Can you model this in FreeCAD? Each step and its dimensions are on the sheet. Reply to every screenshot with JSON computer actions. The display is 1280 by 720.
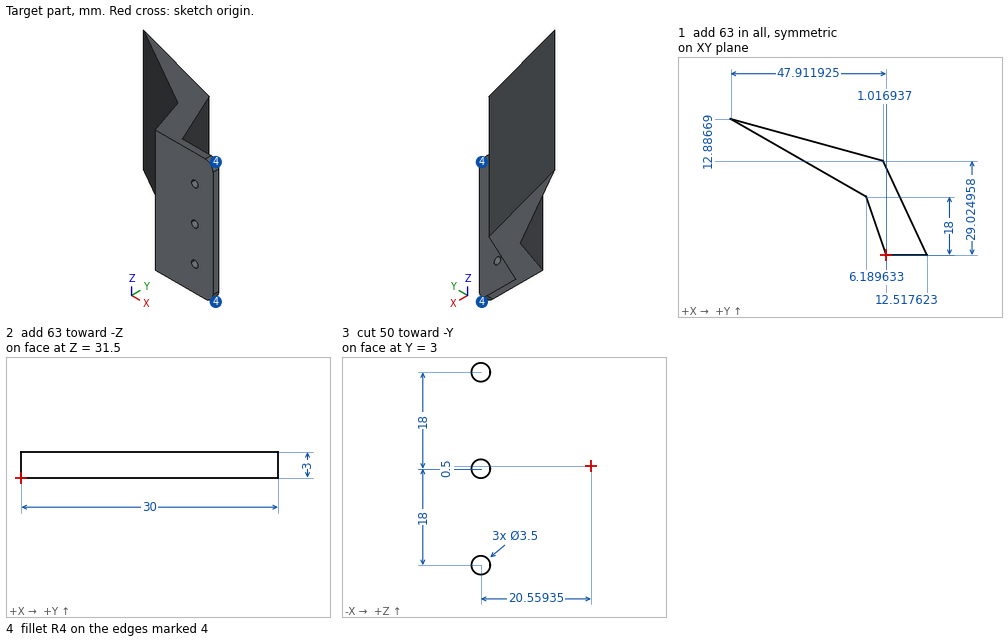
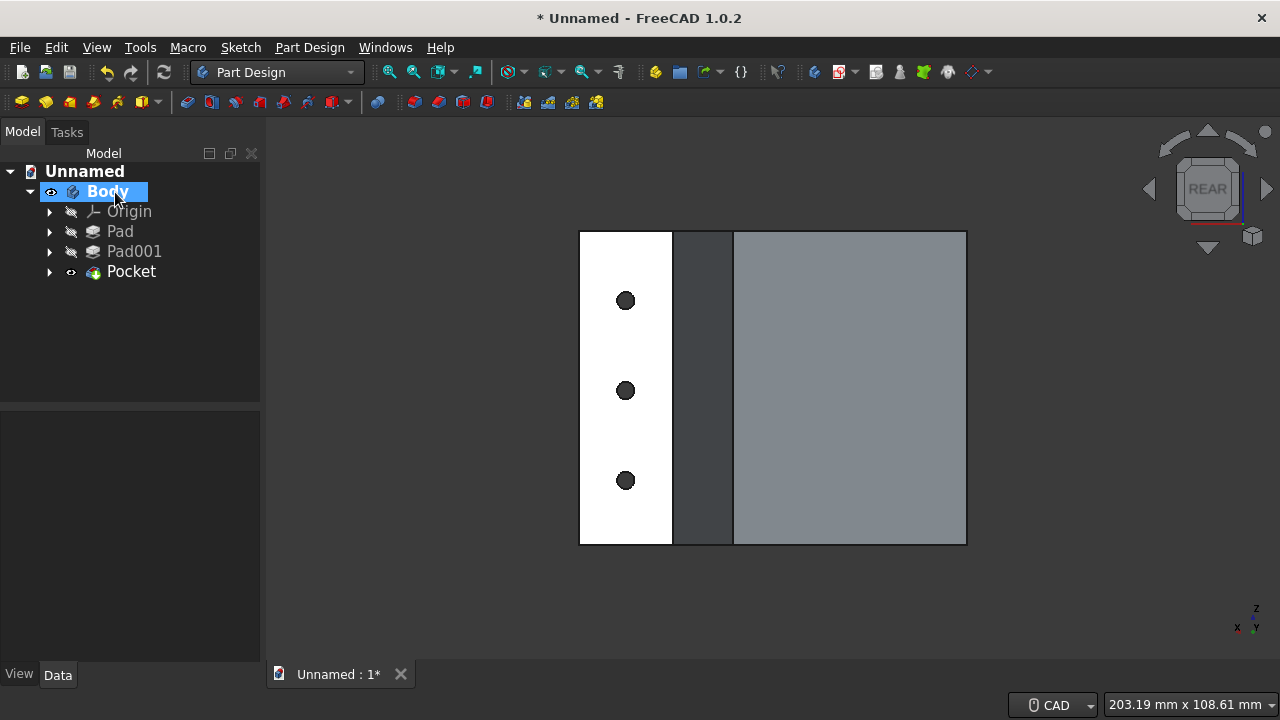
{"action": "scroll", "coordinate": [579, 230], "scroll_direction": "up", "scroll_amount": 5}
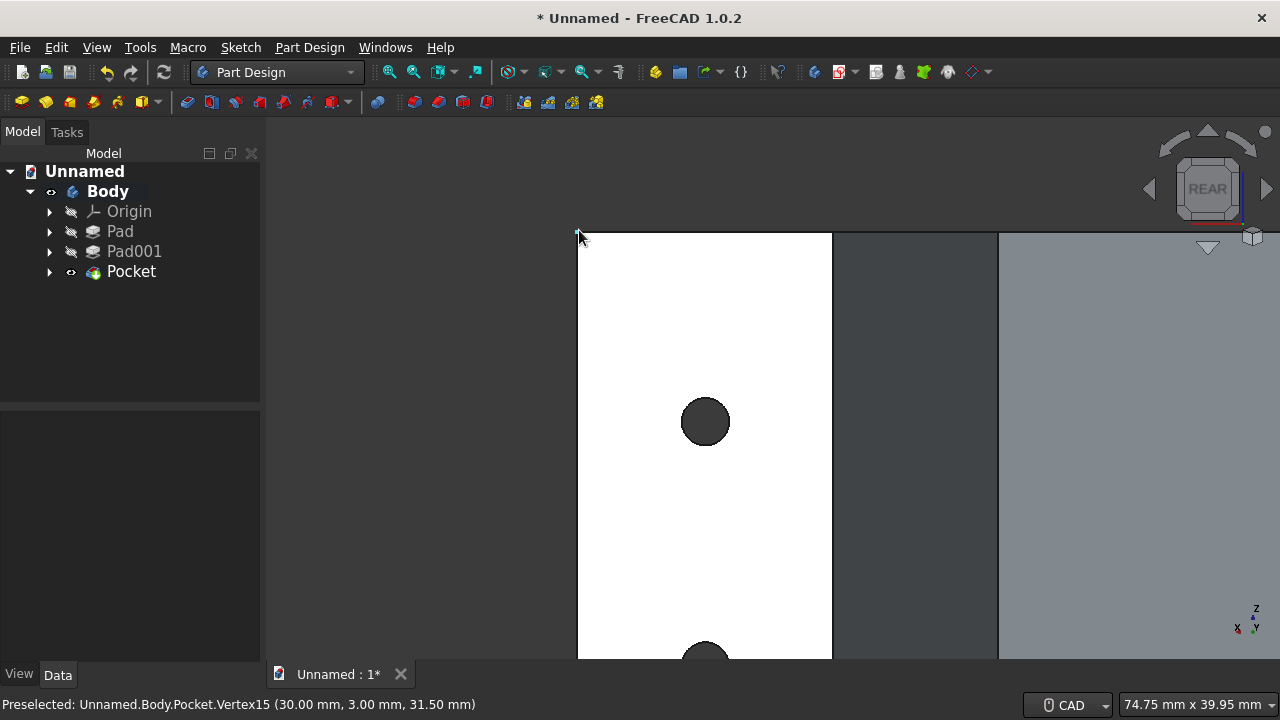
{"action": "key", "text": "v f"}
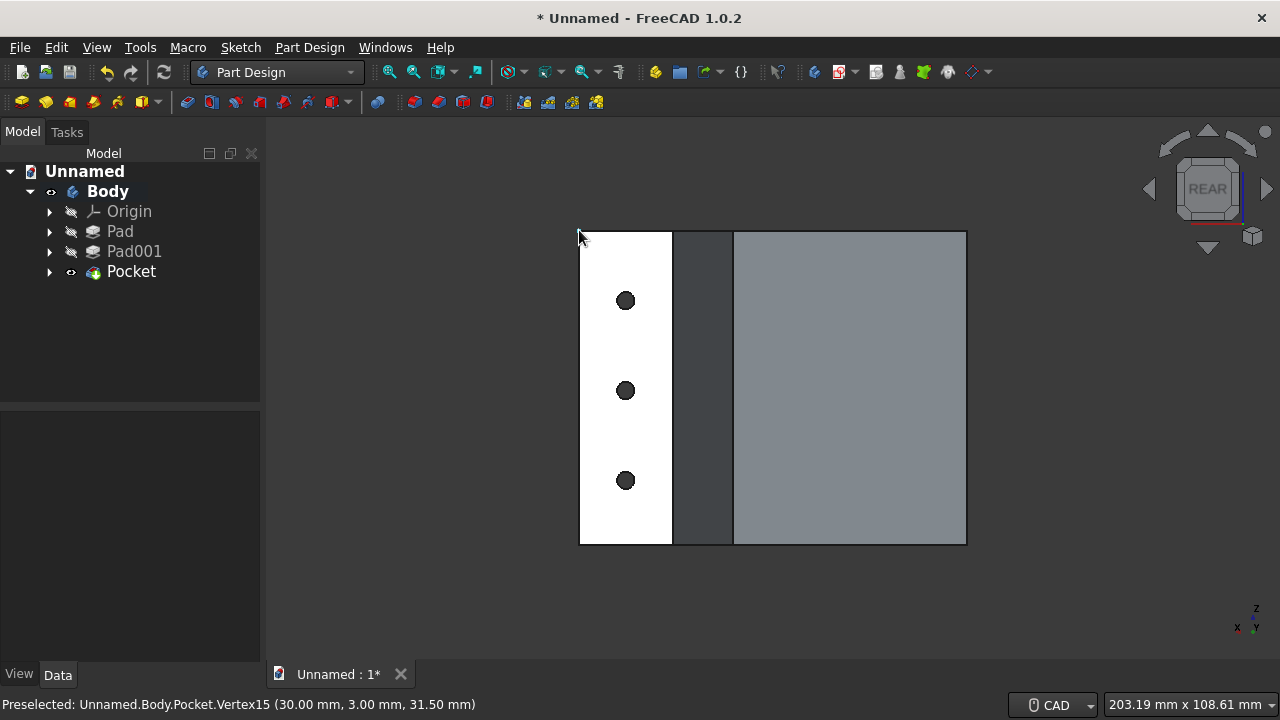
{"action": "key", "text": "0"}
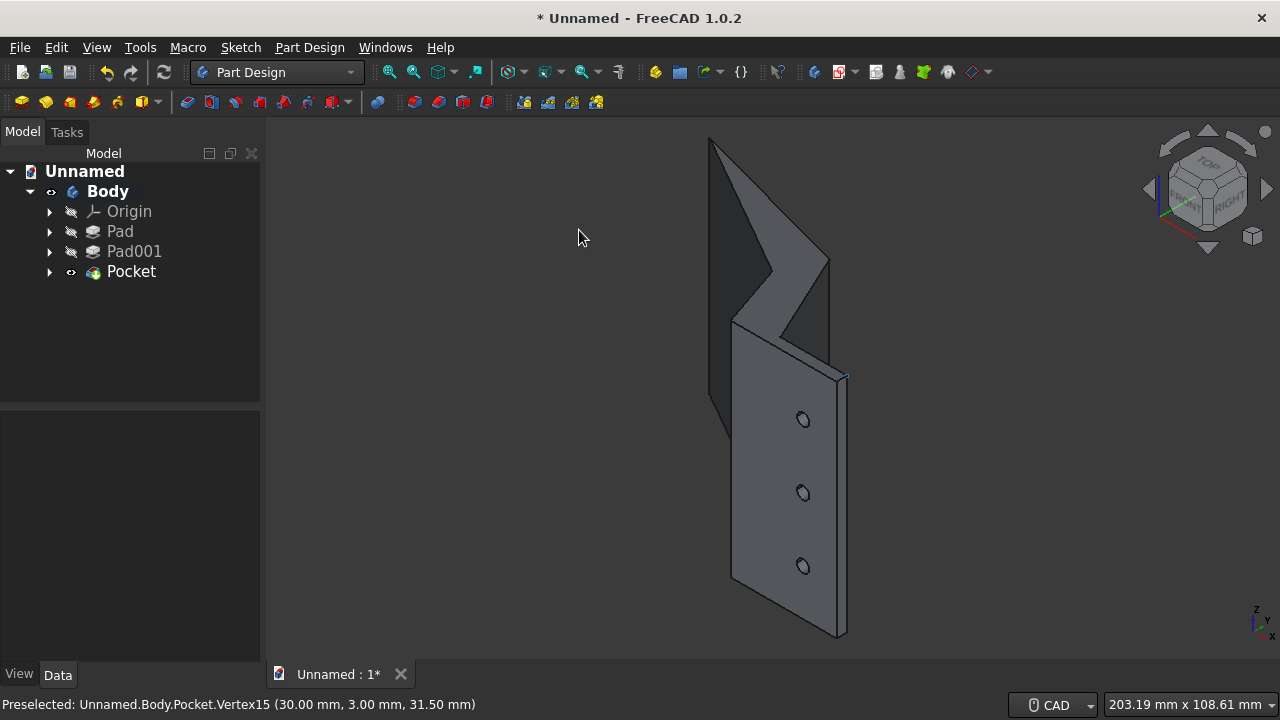
{"action": "left_click", "coordinate": [843, 377]}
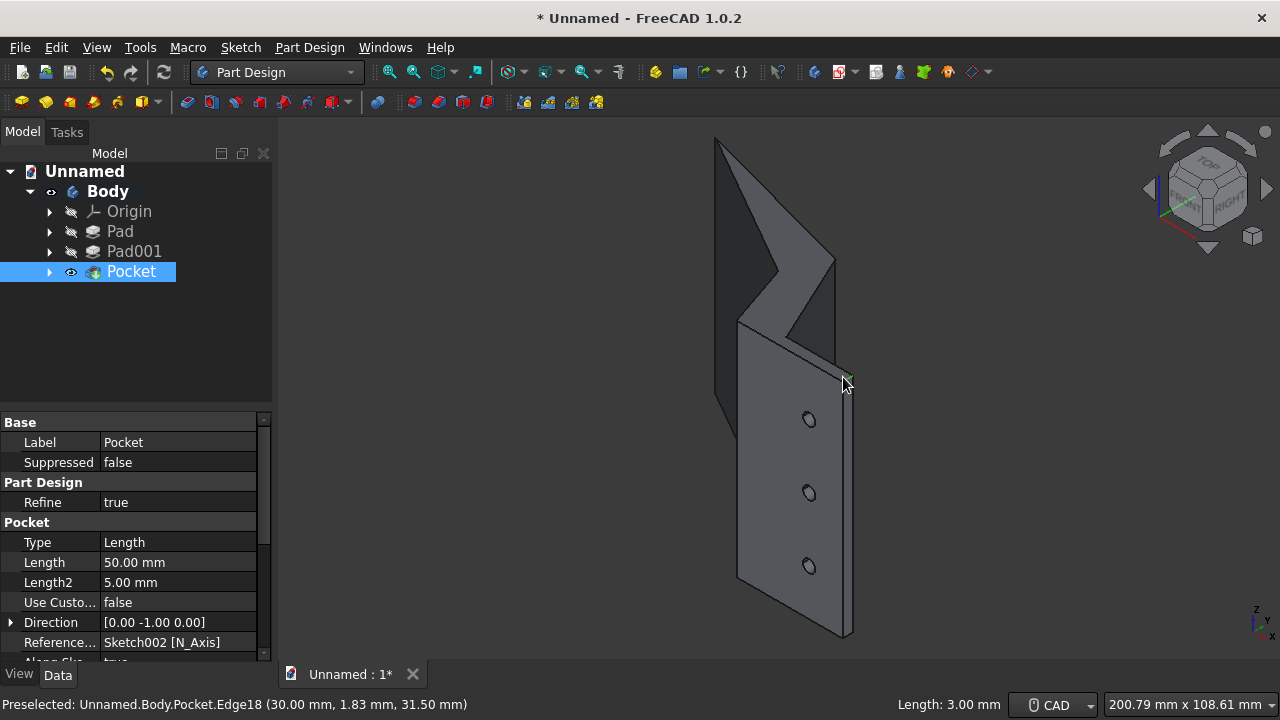
{"action": "key", "text": "2"}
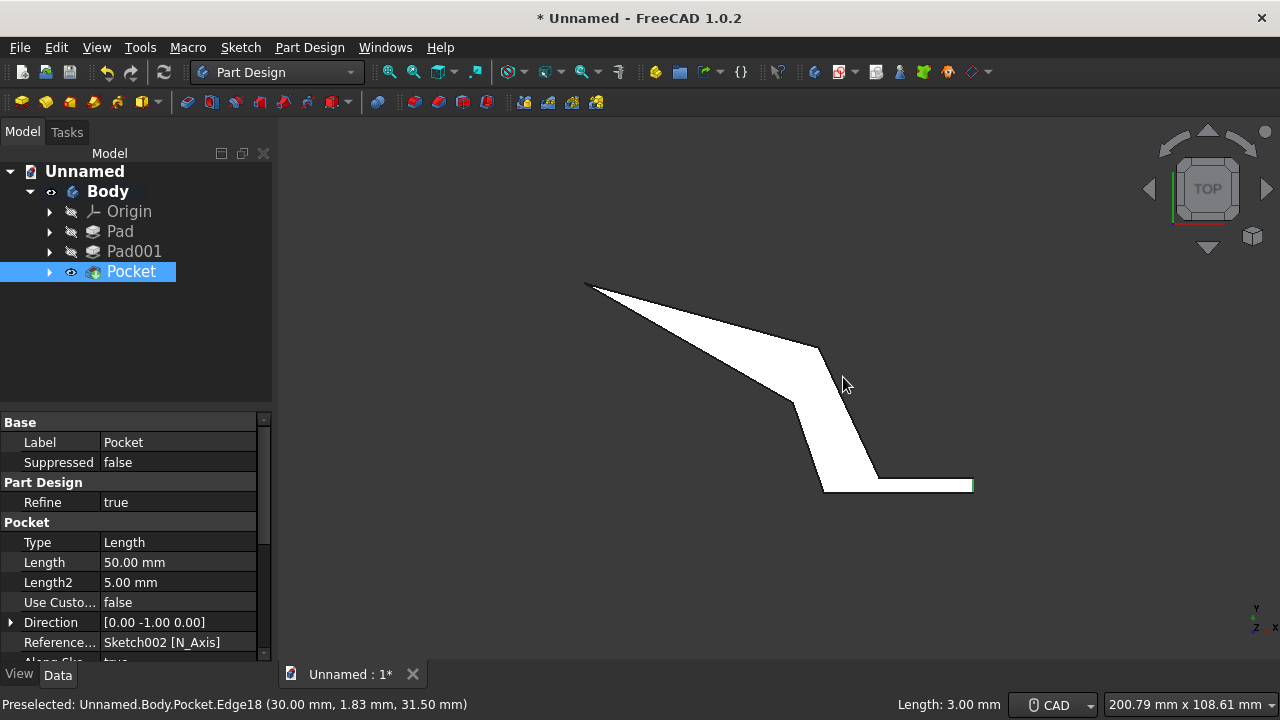
{"action": "key", "text": "v f"}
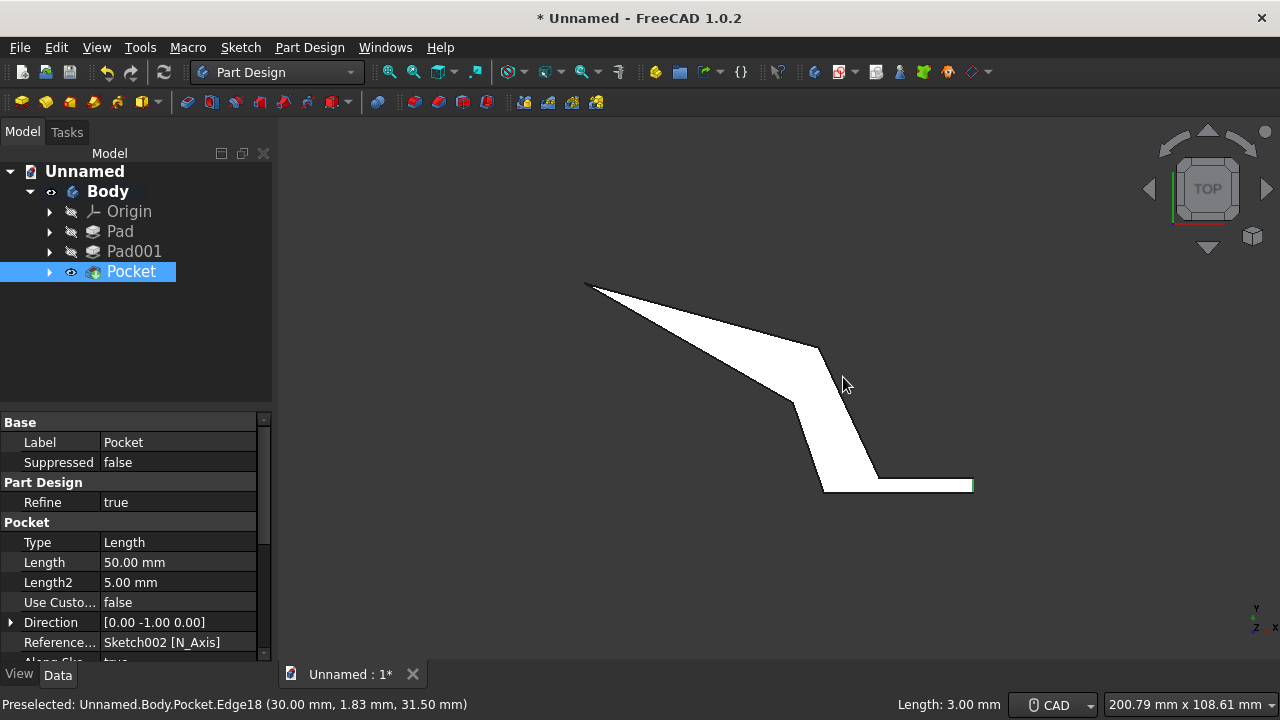
{"action": "scroll", "coordinate": [973, 484], "scroll_direction": "up", "scroll_amount": 5}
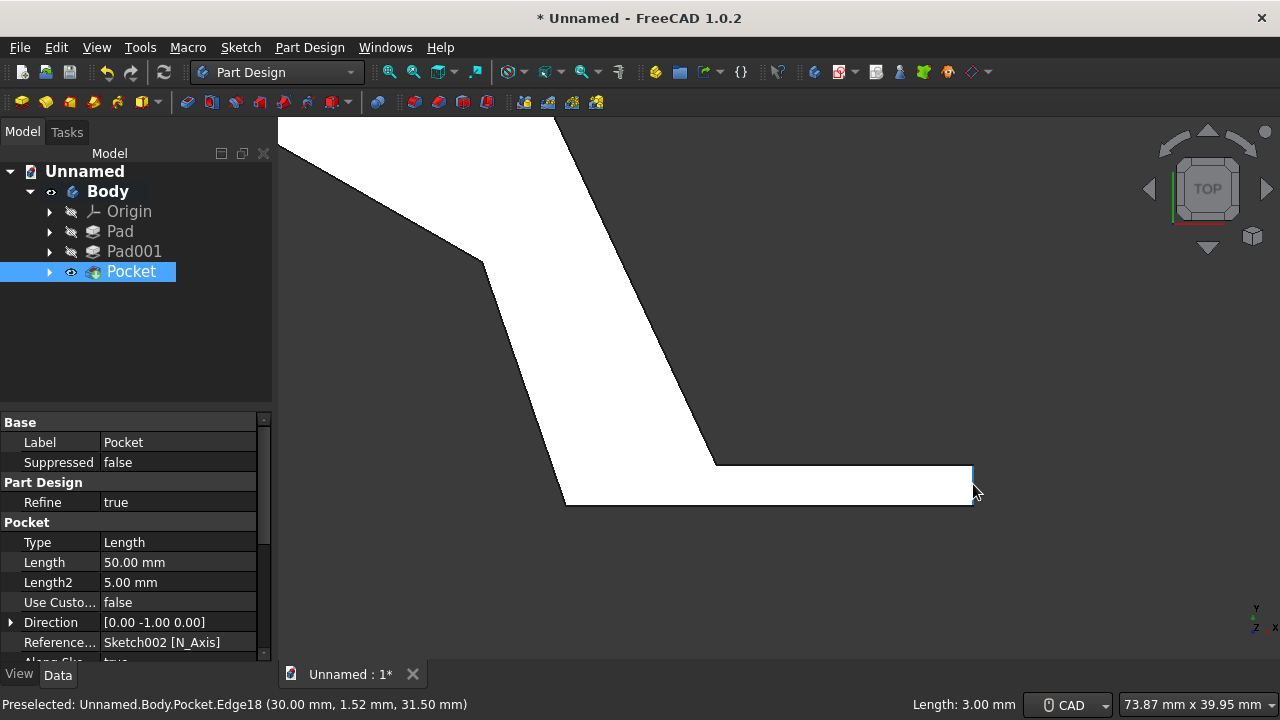
{"action": "key", "text": "v f"}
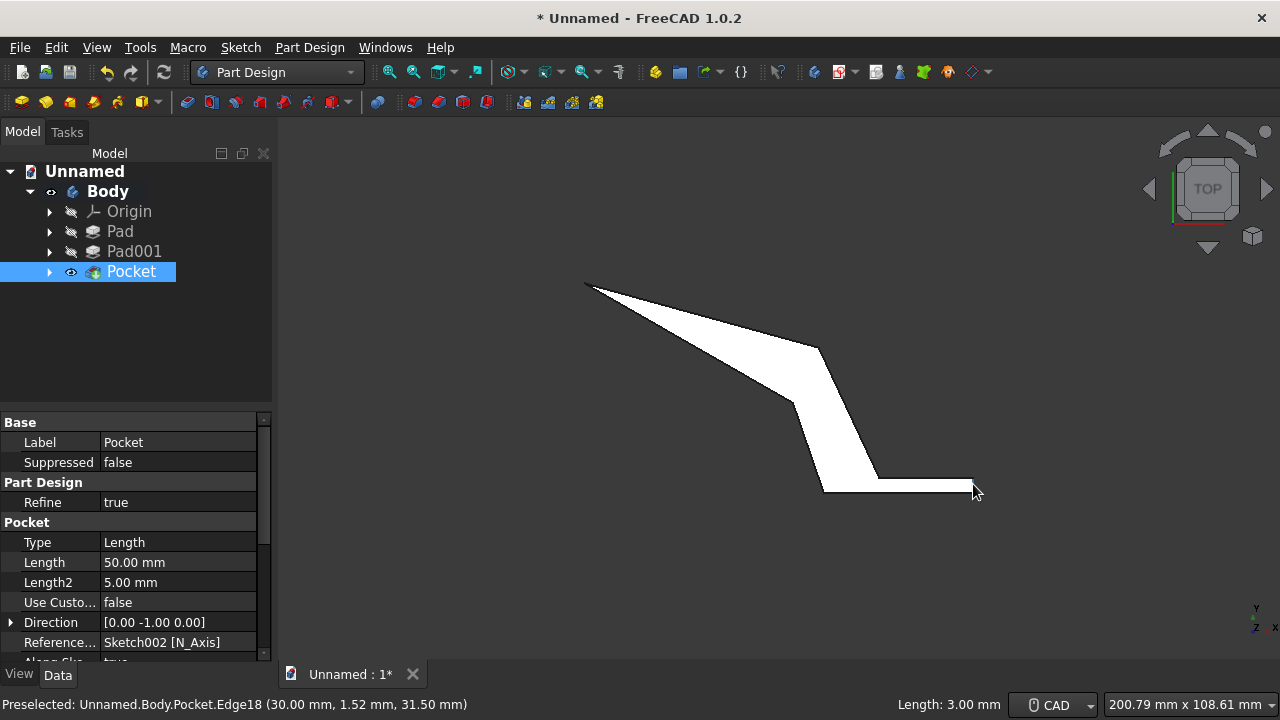
{"action": "key", "text": "1"}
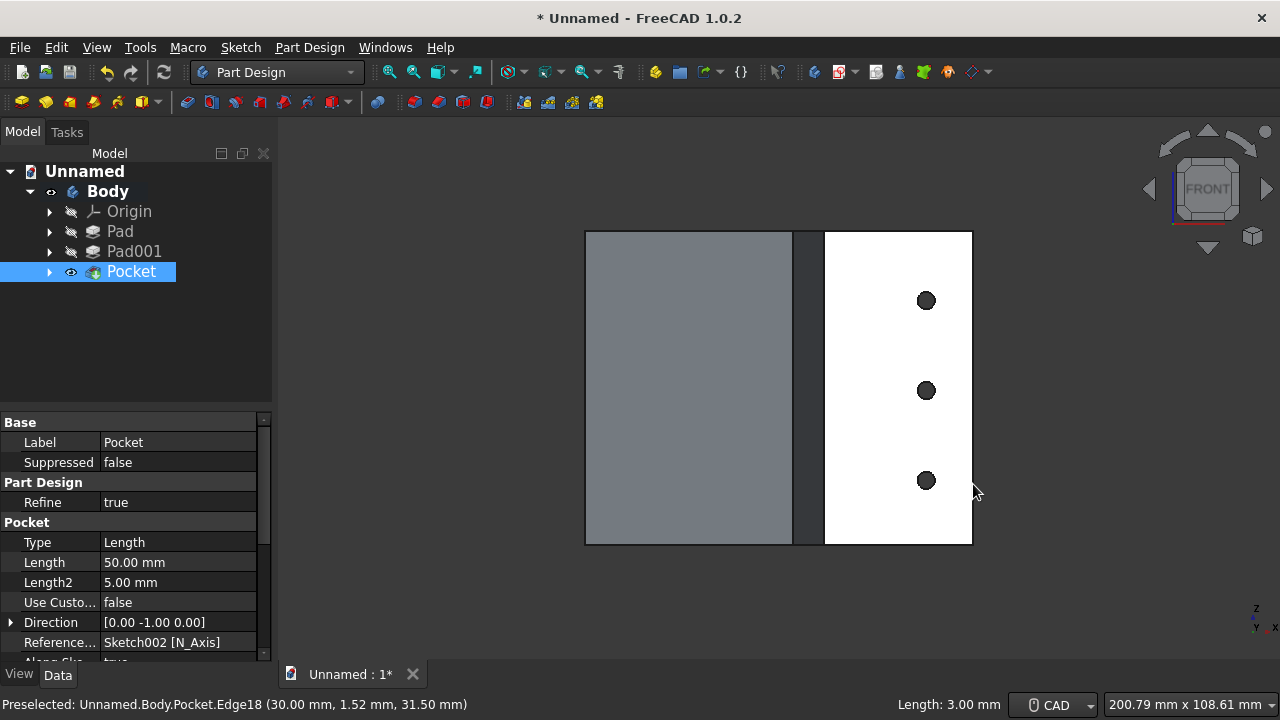
{"action": "scroll", "coordinate": [973, 544], "scroll_direction": "up", "scroll_amount": 5}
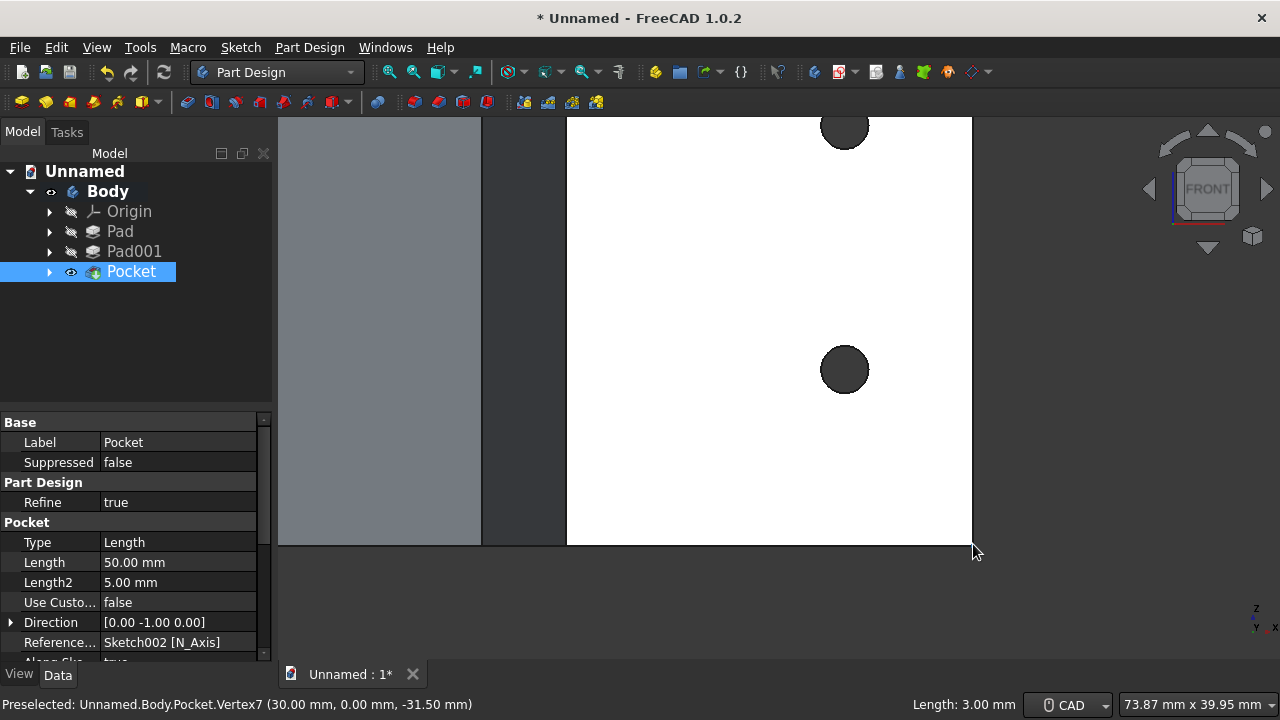
{"action": "key", "text": "v f"}